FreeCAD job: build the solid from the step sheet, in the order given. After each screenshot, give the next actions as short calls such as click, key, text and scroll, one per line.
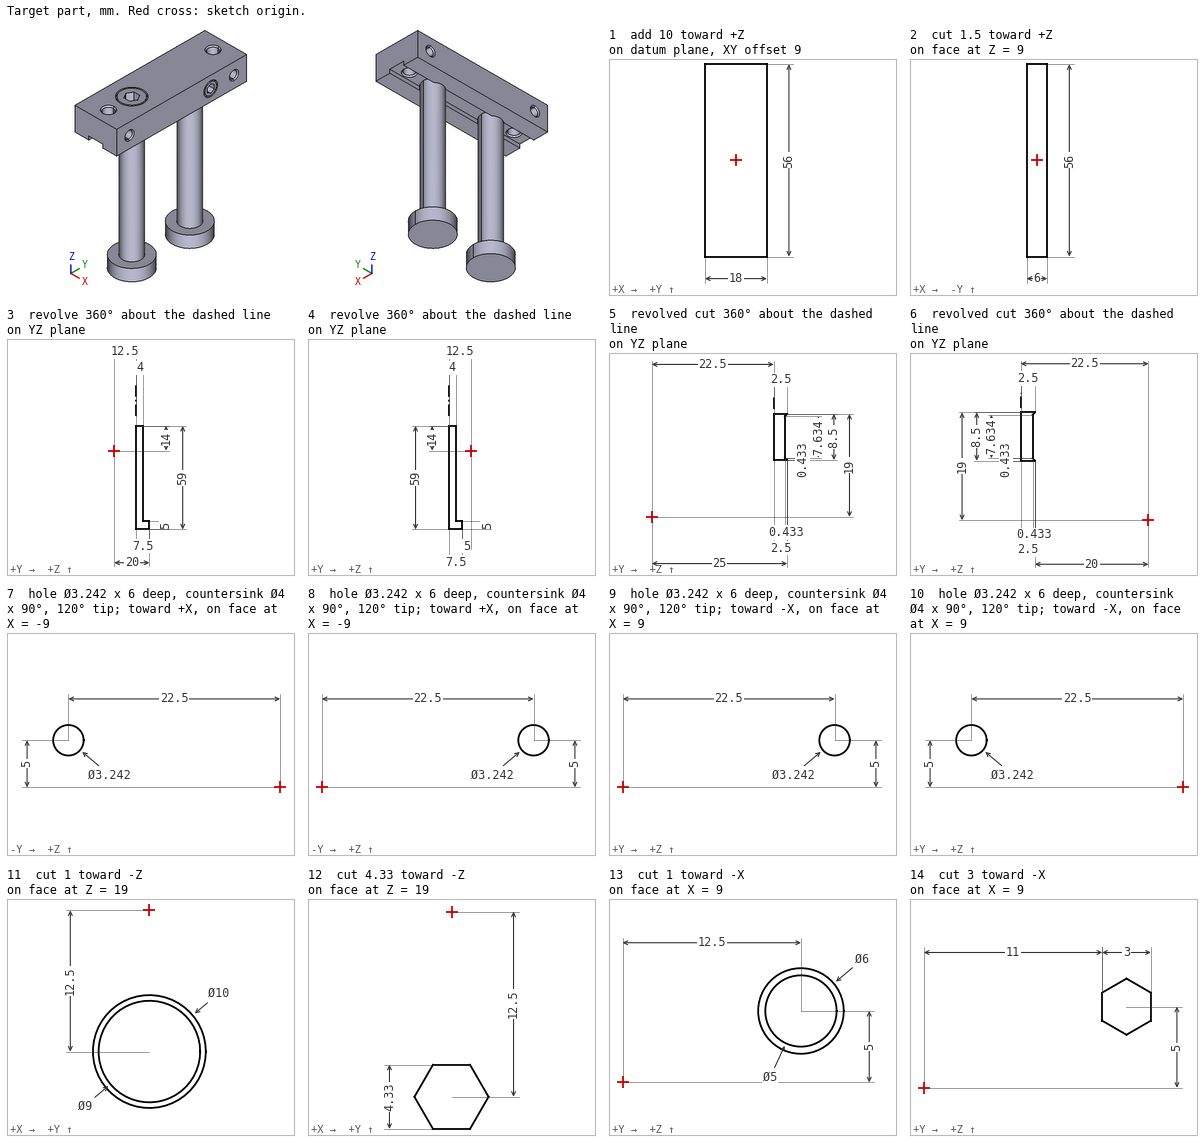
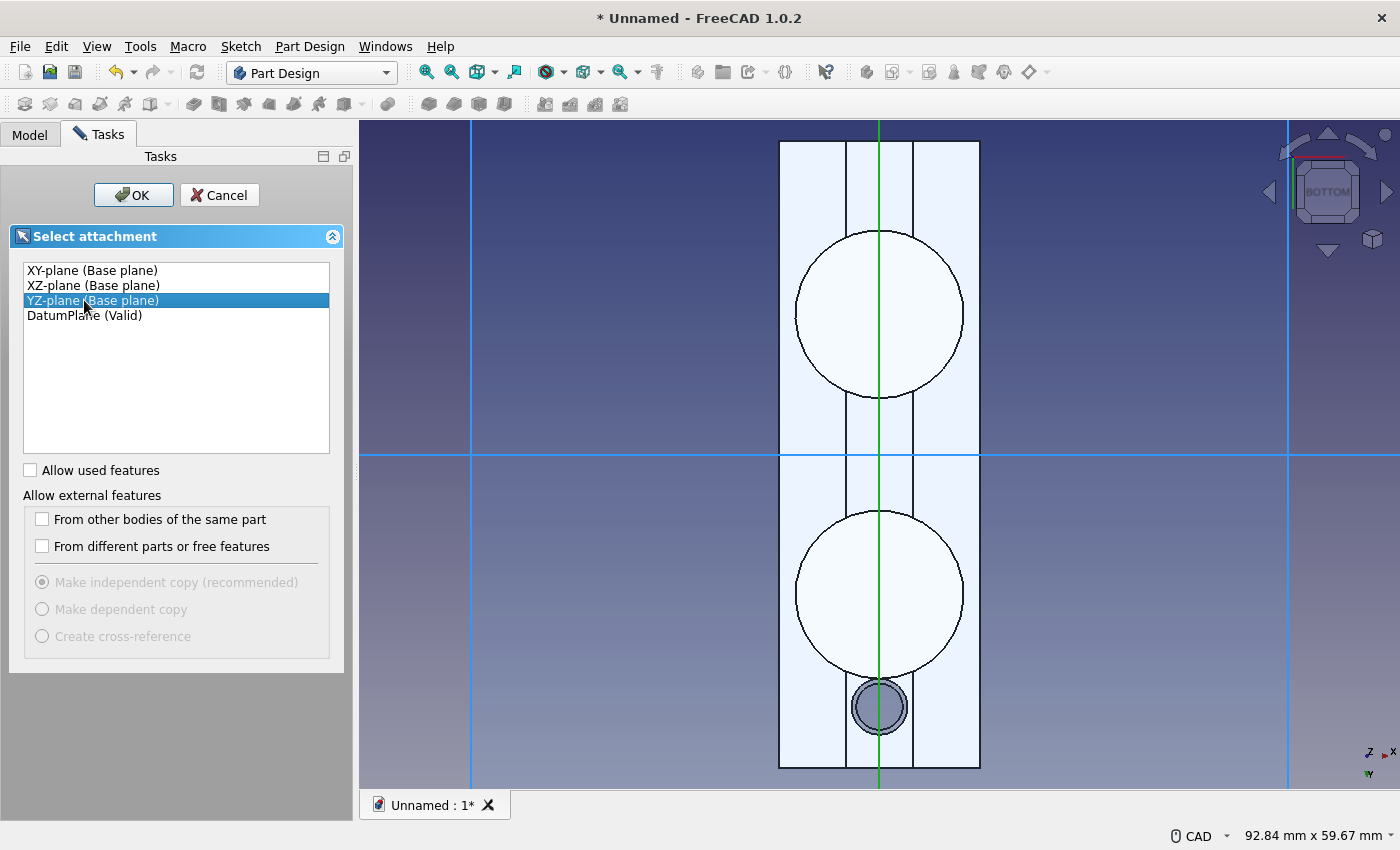
click(134, 195)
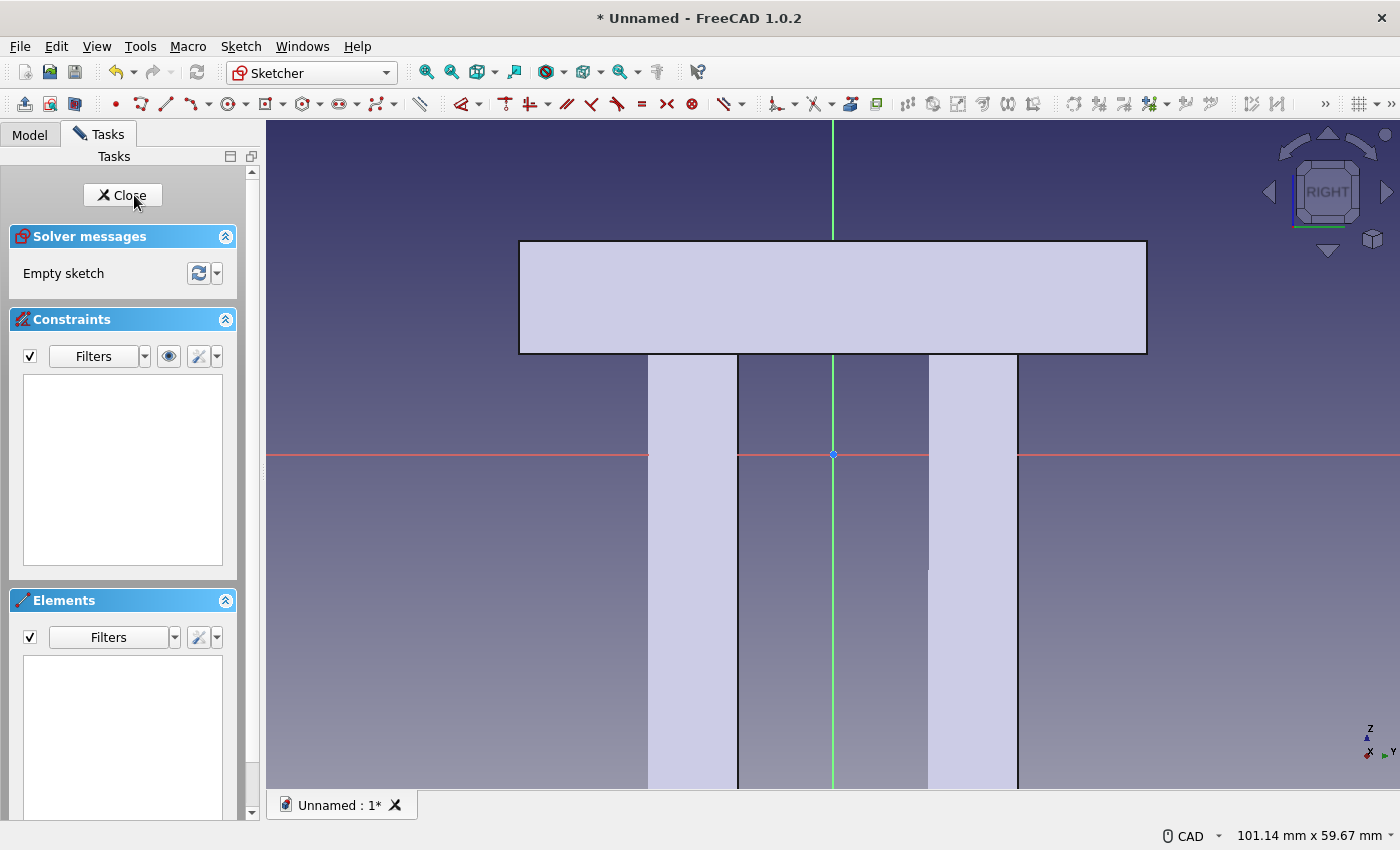
click(75, 104)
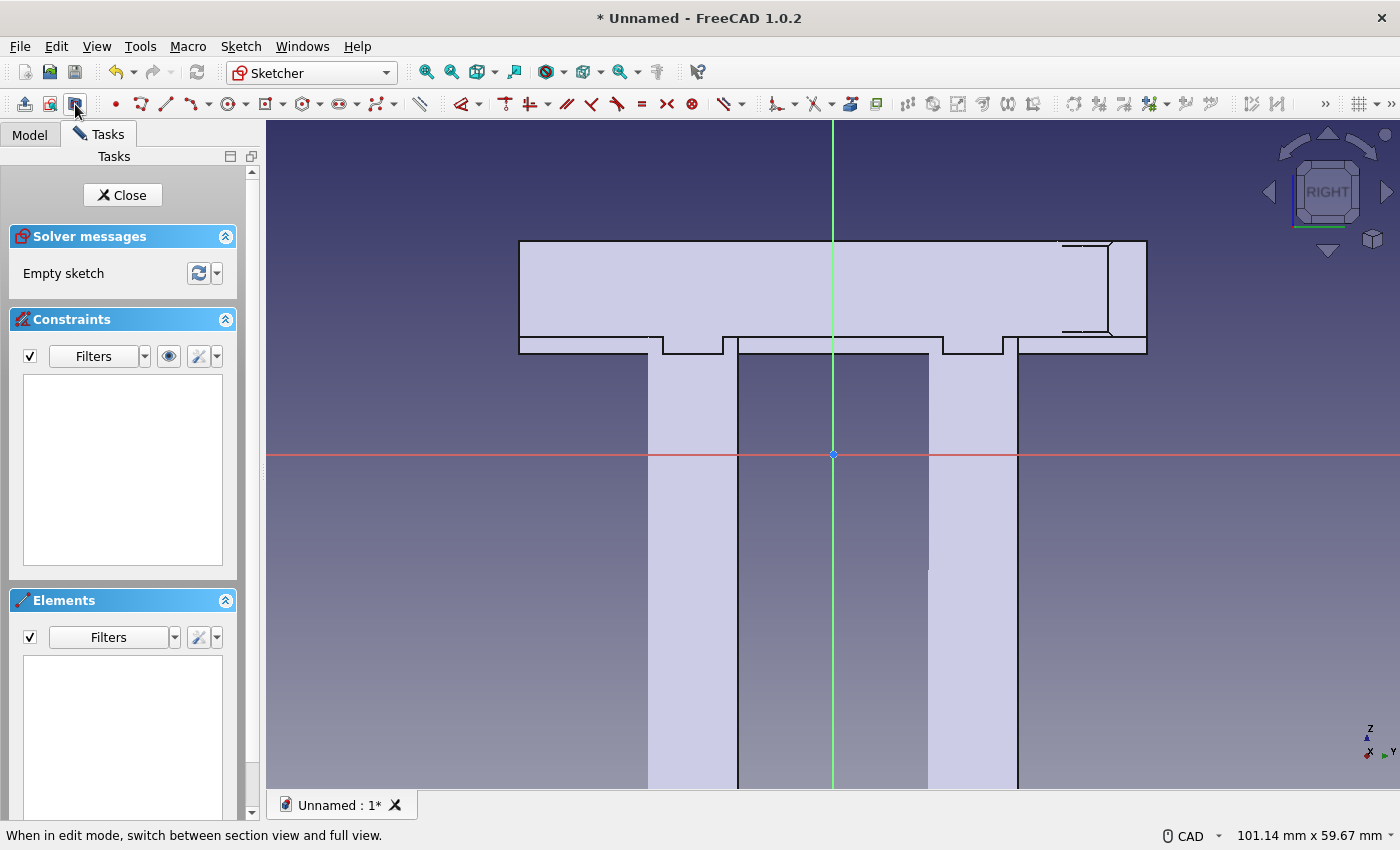
scroll(637, 176, up, 3)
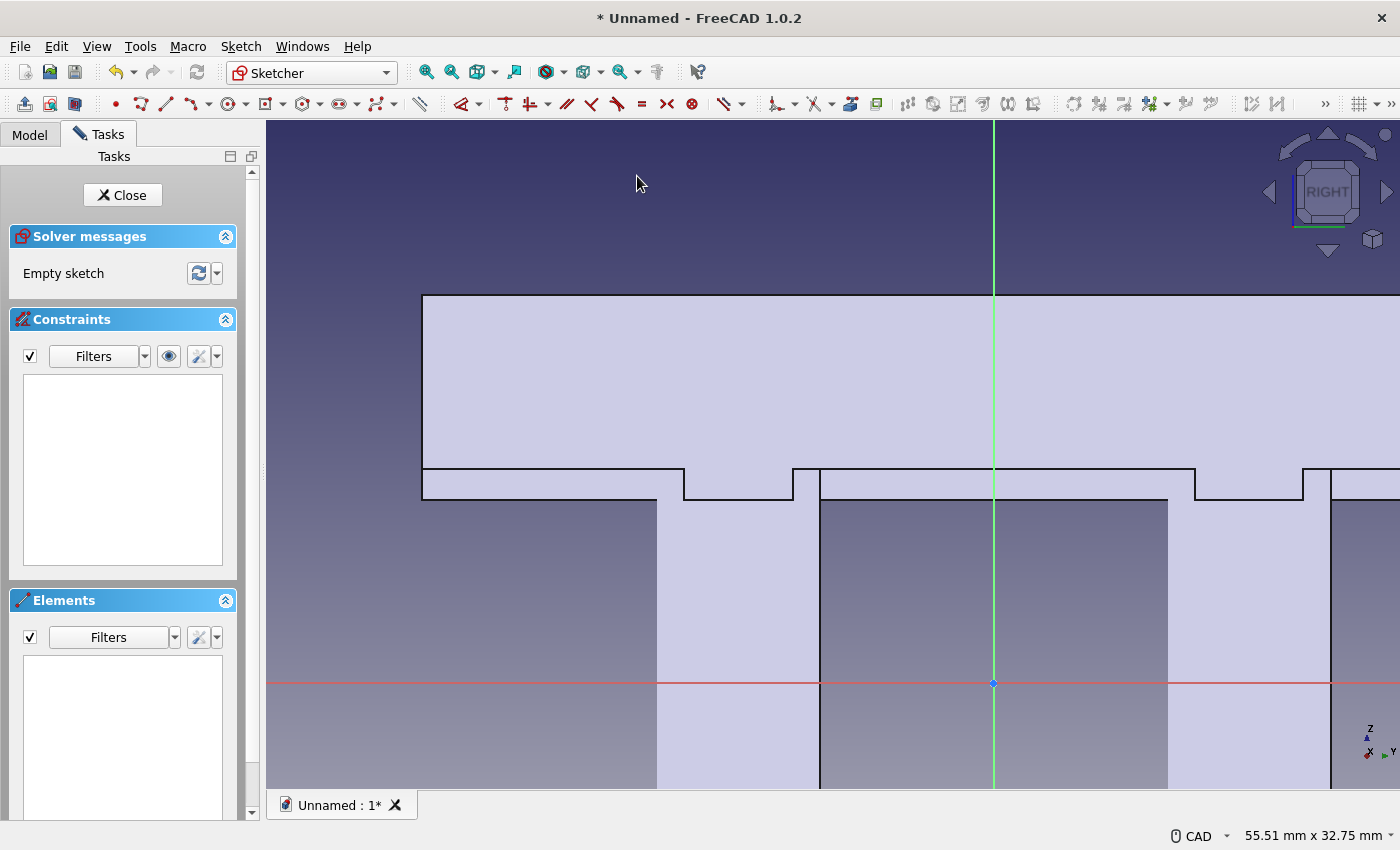
click(141, 104)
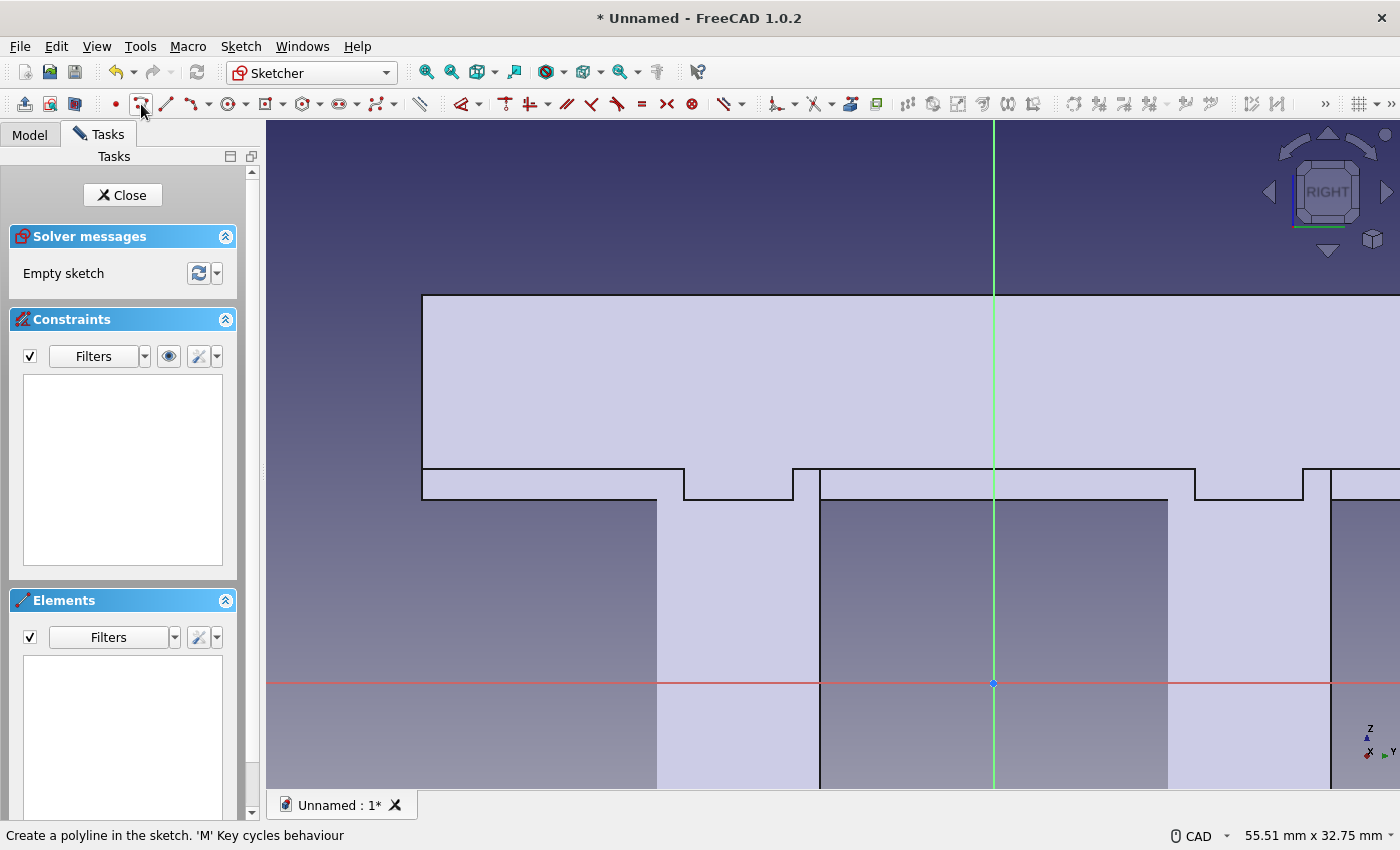
click(585, 469)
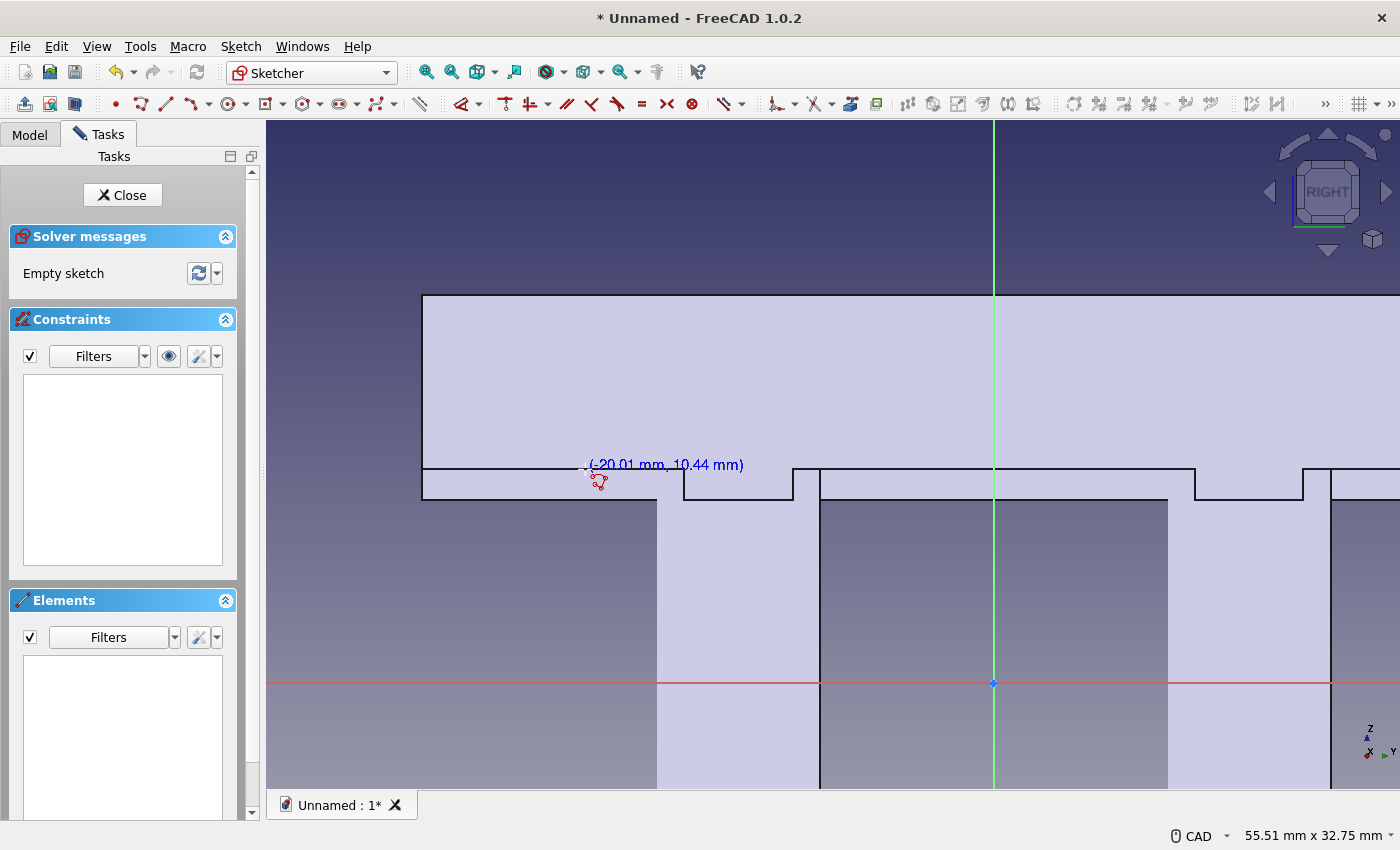
scroll(576, 460, up, 2)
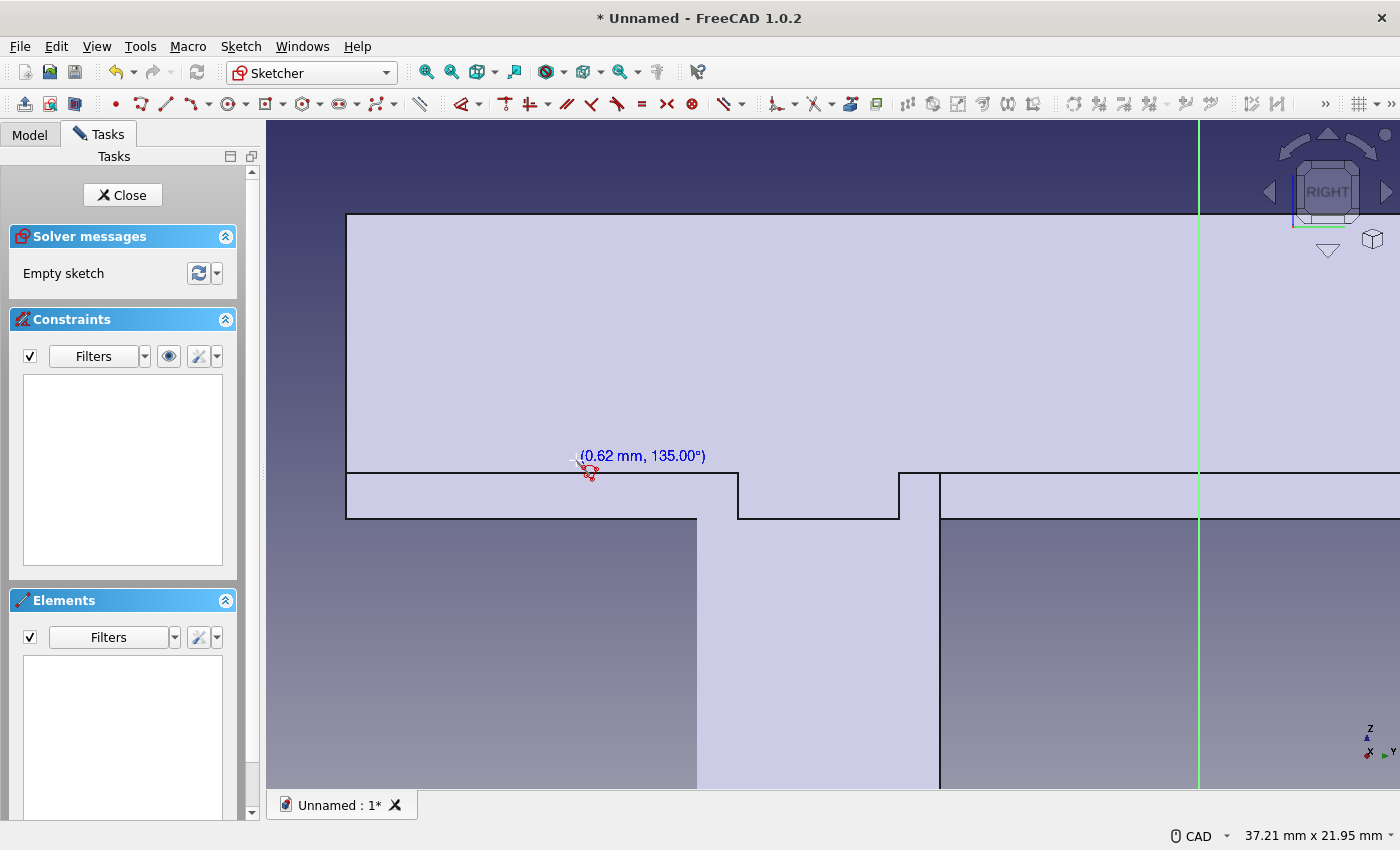
click(576, 460)
click(576, 227)
click(590, 214)
click(513, 214)
click(513, 473)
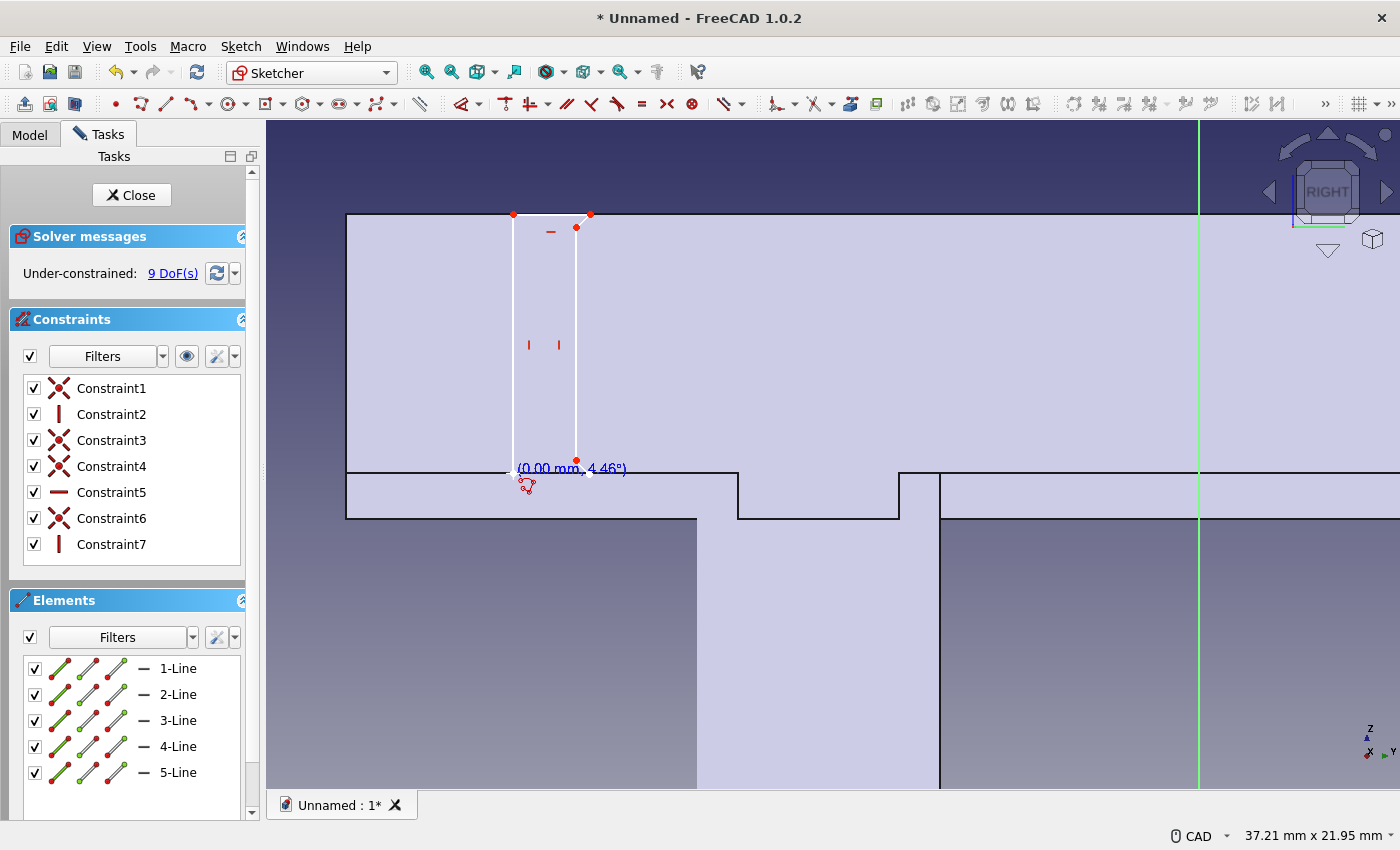
scroll(590, 473, up, 3)